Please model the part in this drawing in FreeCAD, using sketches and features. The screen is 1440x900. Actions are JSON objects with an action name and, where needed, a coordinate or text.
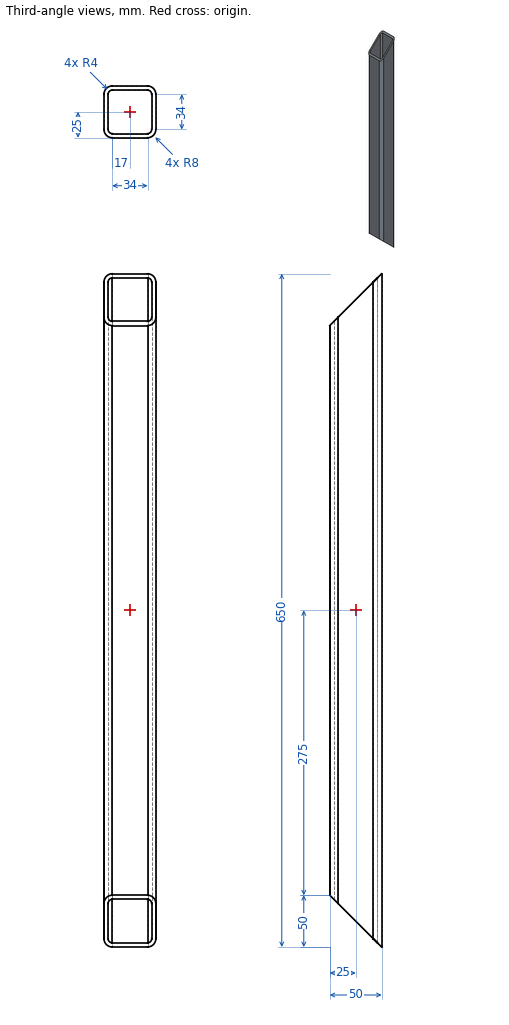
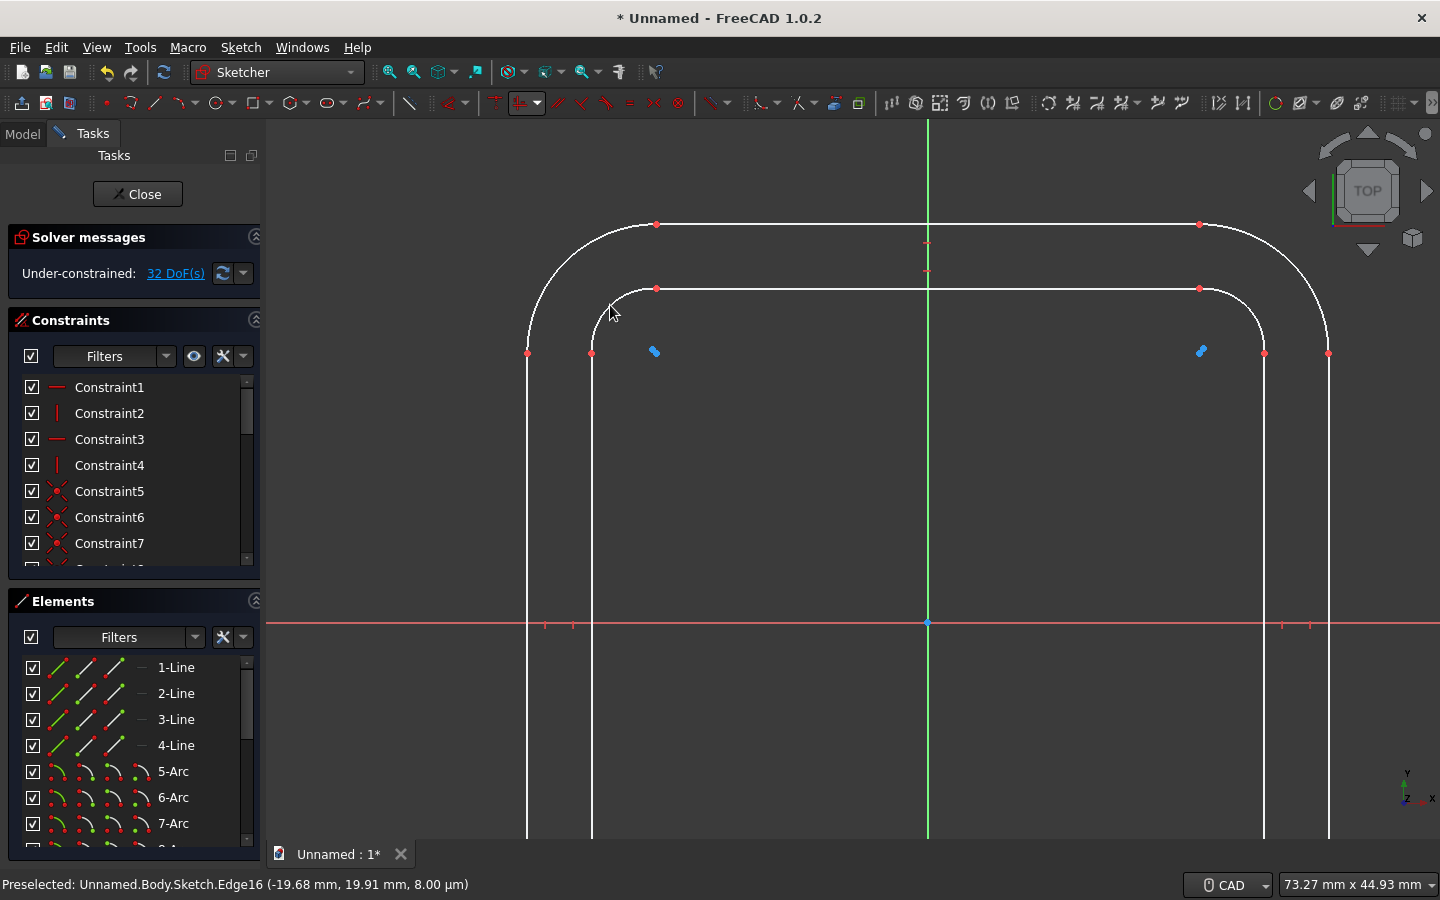
{"action": "scroll", "coordinate": [610, 304], "scroll_direction": "down", "scroll_amount": 3}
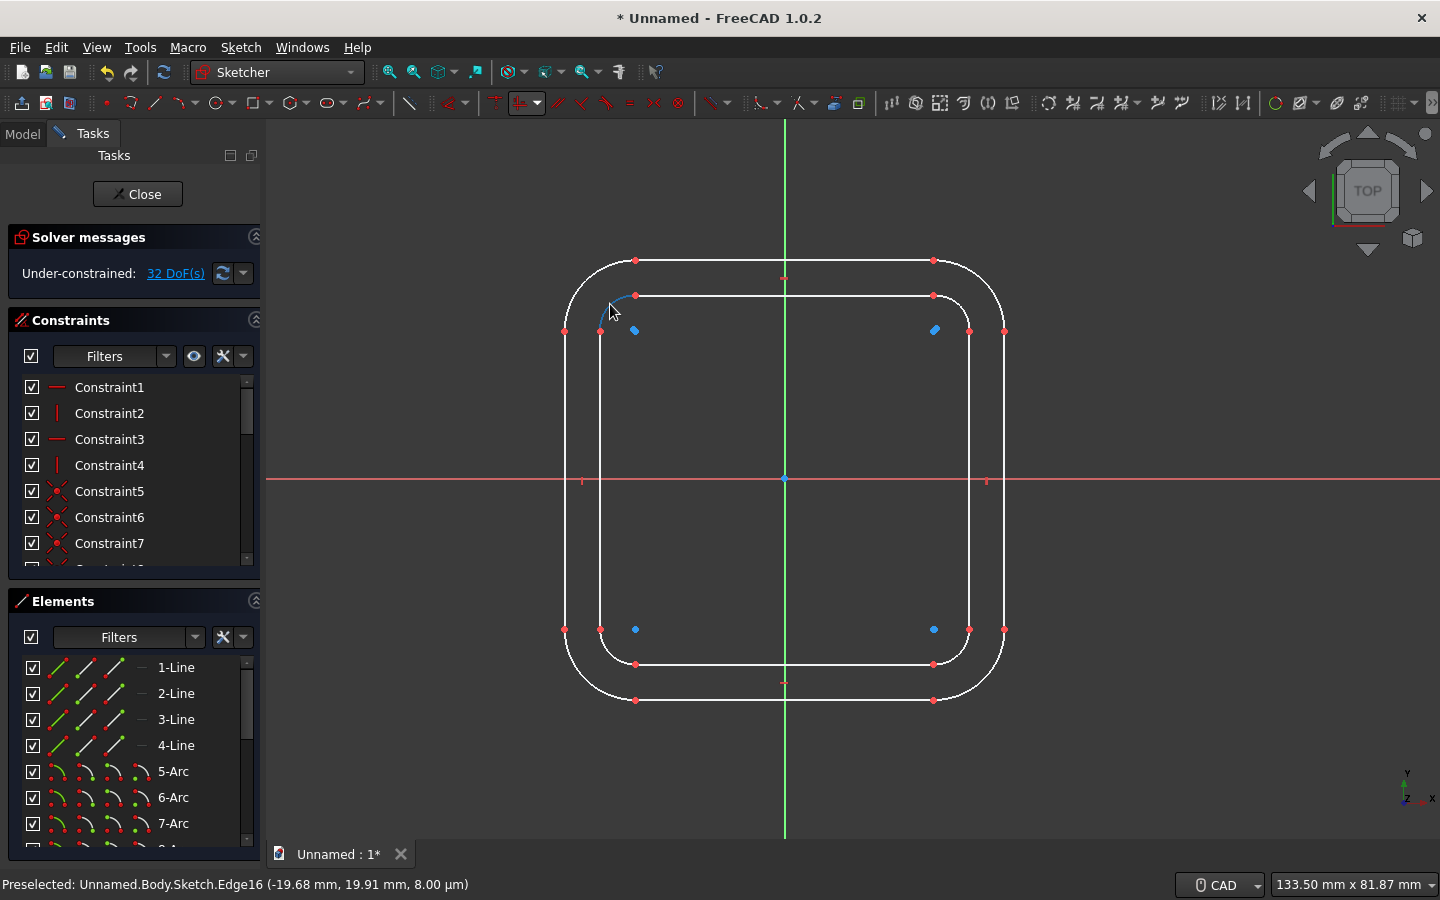
{"action": "left_click", "coordinate": [725, 700]}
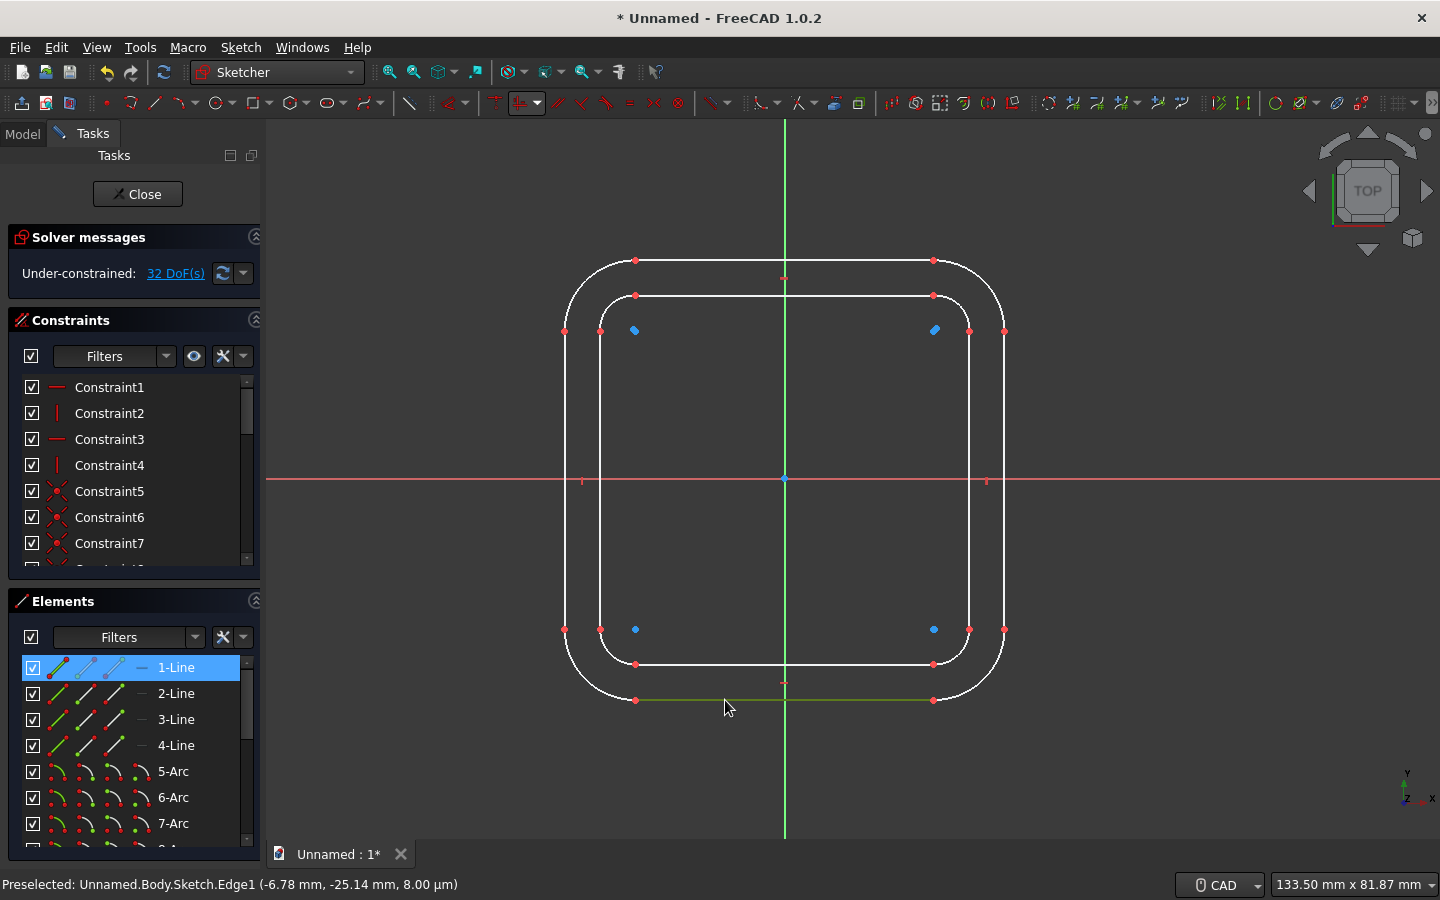
{"action": "left_click", "coordinate": [966, 692]}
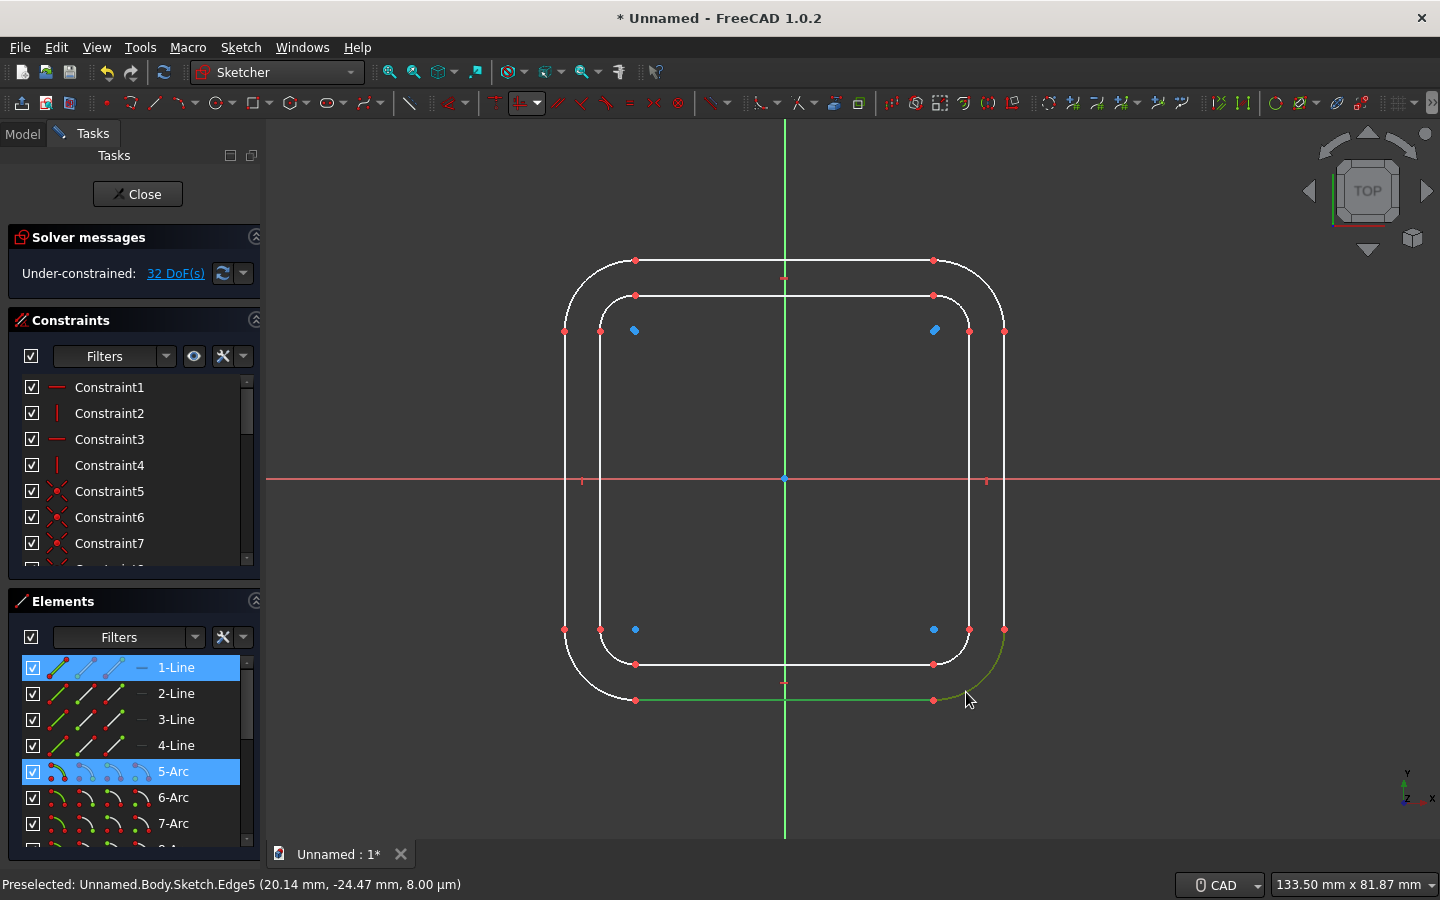
{"action": "left_click", "coordinate": [606, 104]}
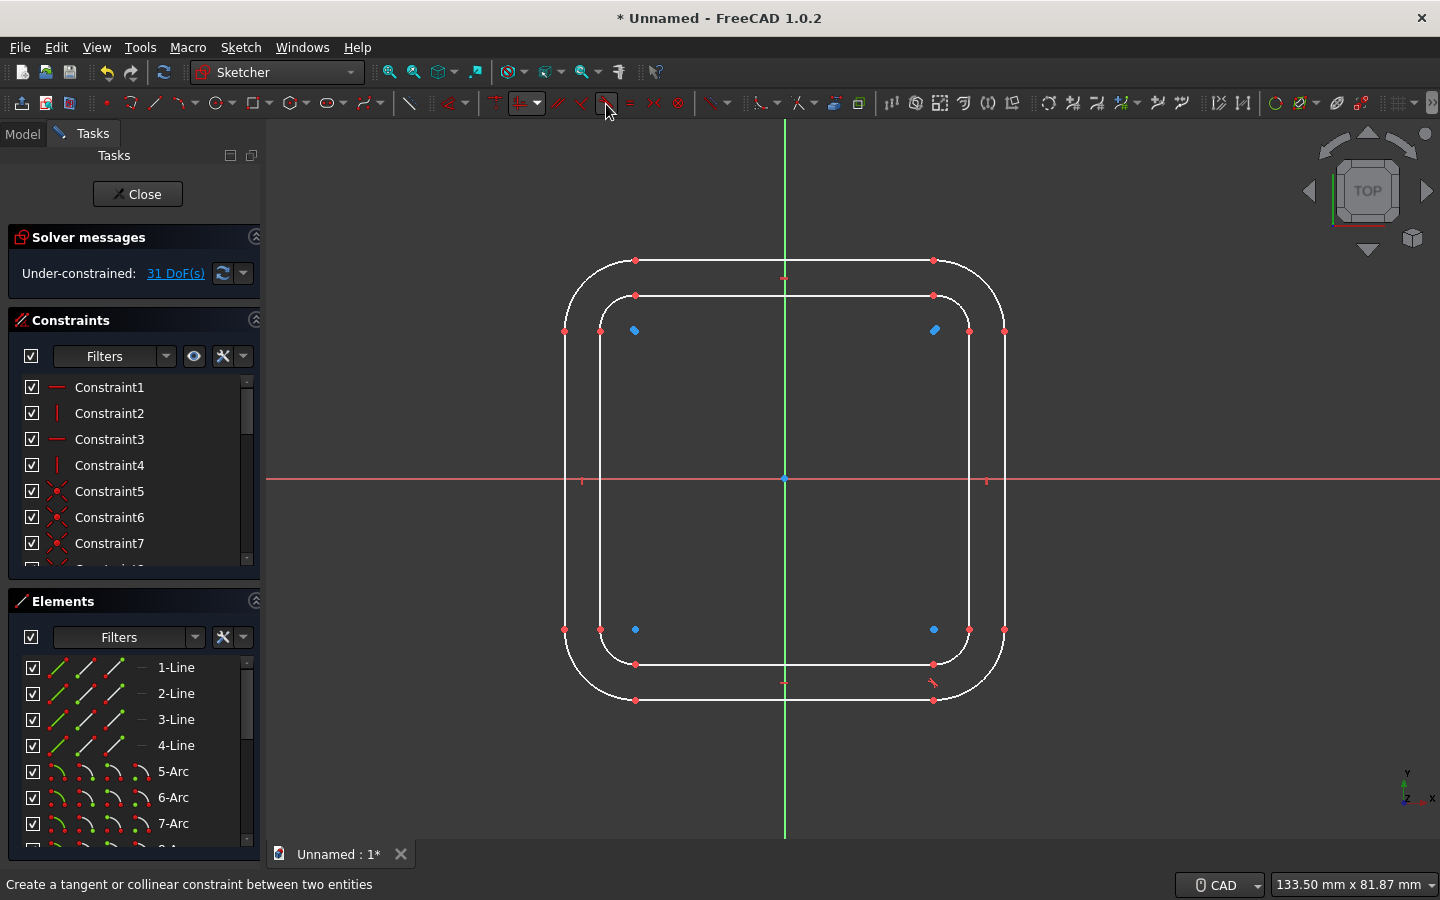
{"action": "left_click", "coordinate": [725, 700]}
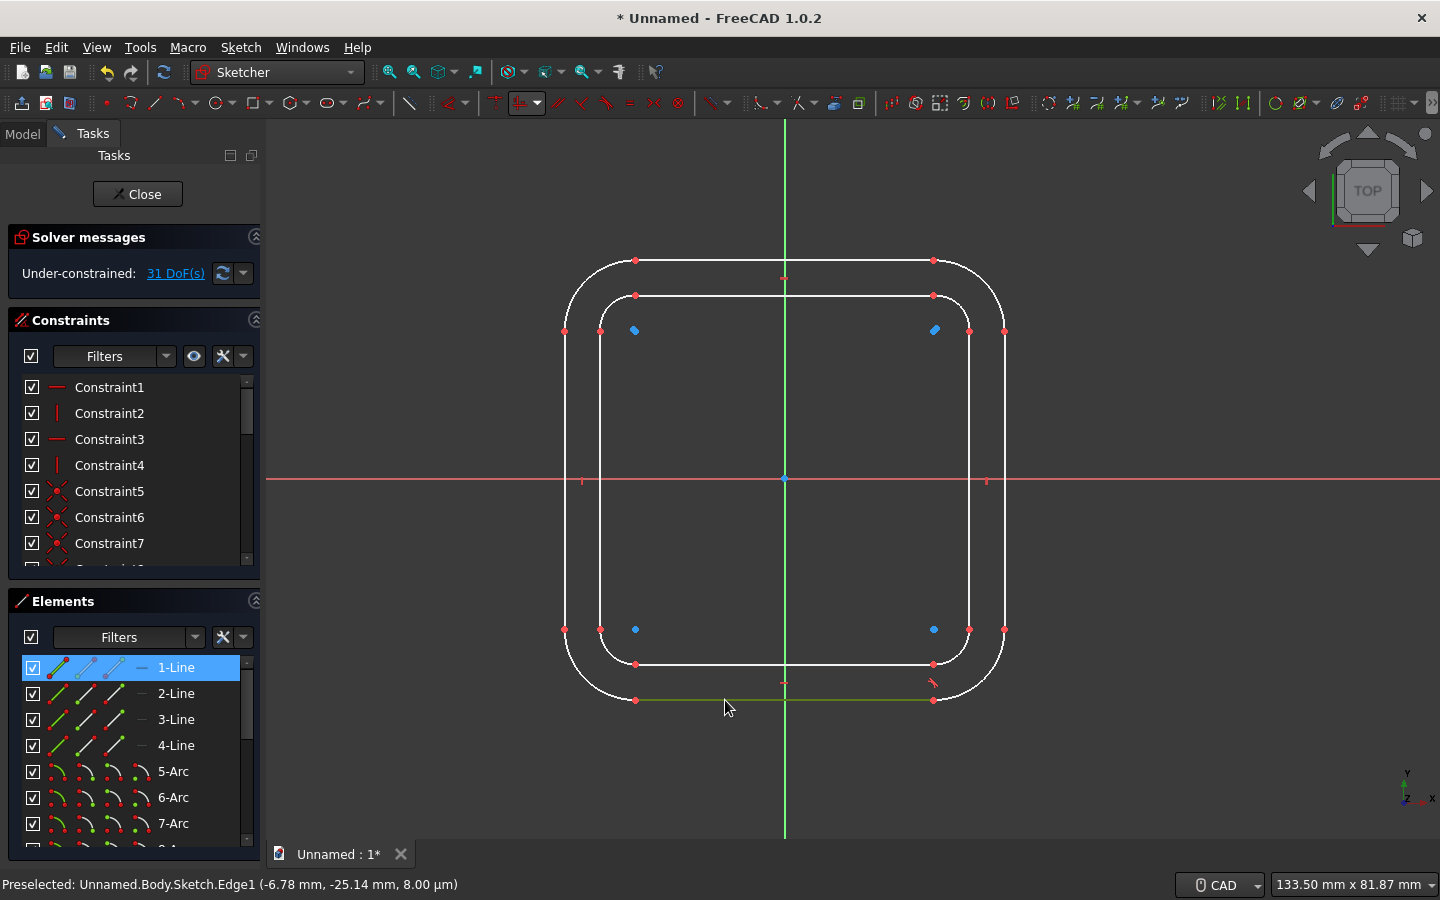
{"action": "left_click", "coordinate": [573, 661]}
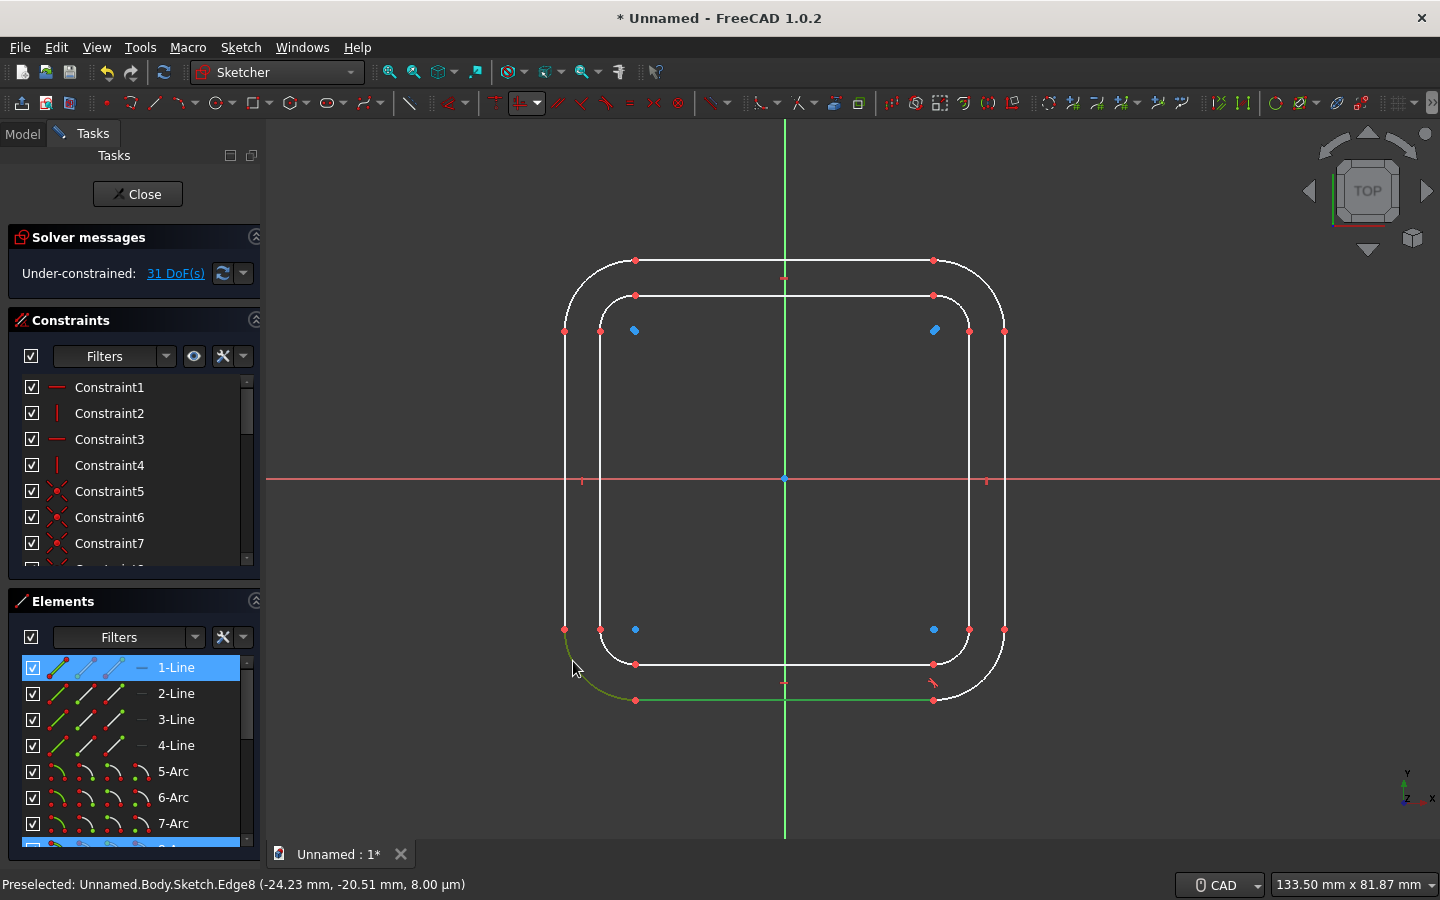
{"action": "left_click", "coordinate": [606, 104]}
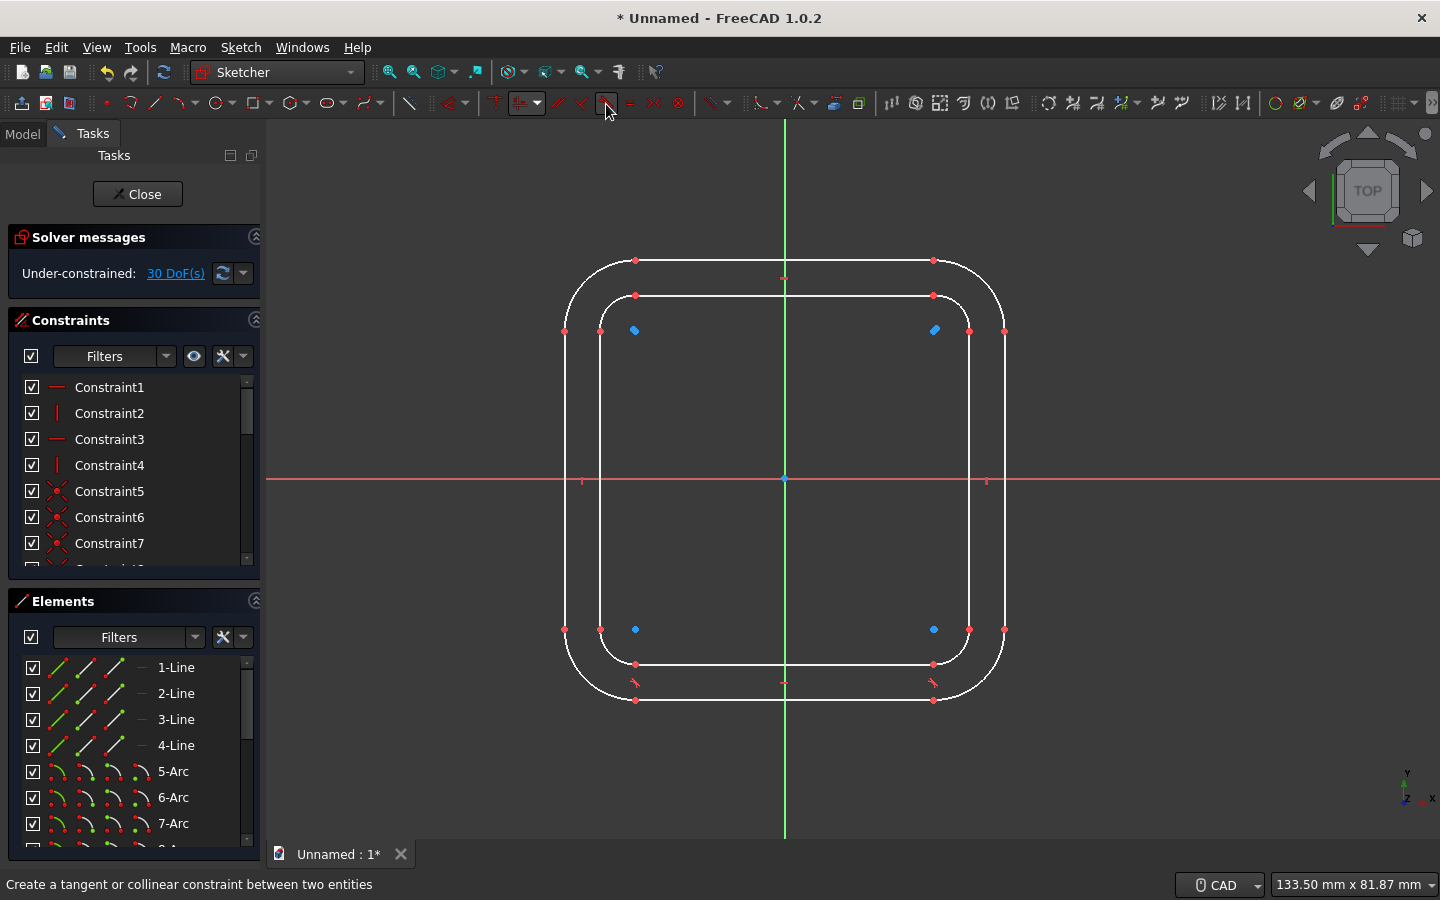
{"action": "left_click", "coordinate": [1005, 540]}